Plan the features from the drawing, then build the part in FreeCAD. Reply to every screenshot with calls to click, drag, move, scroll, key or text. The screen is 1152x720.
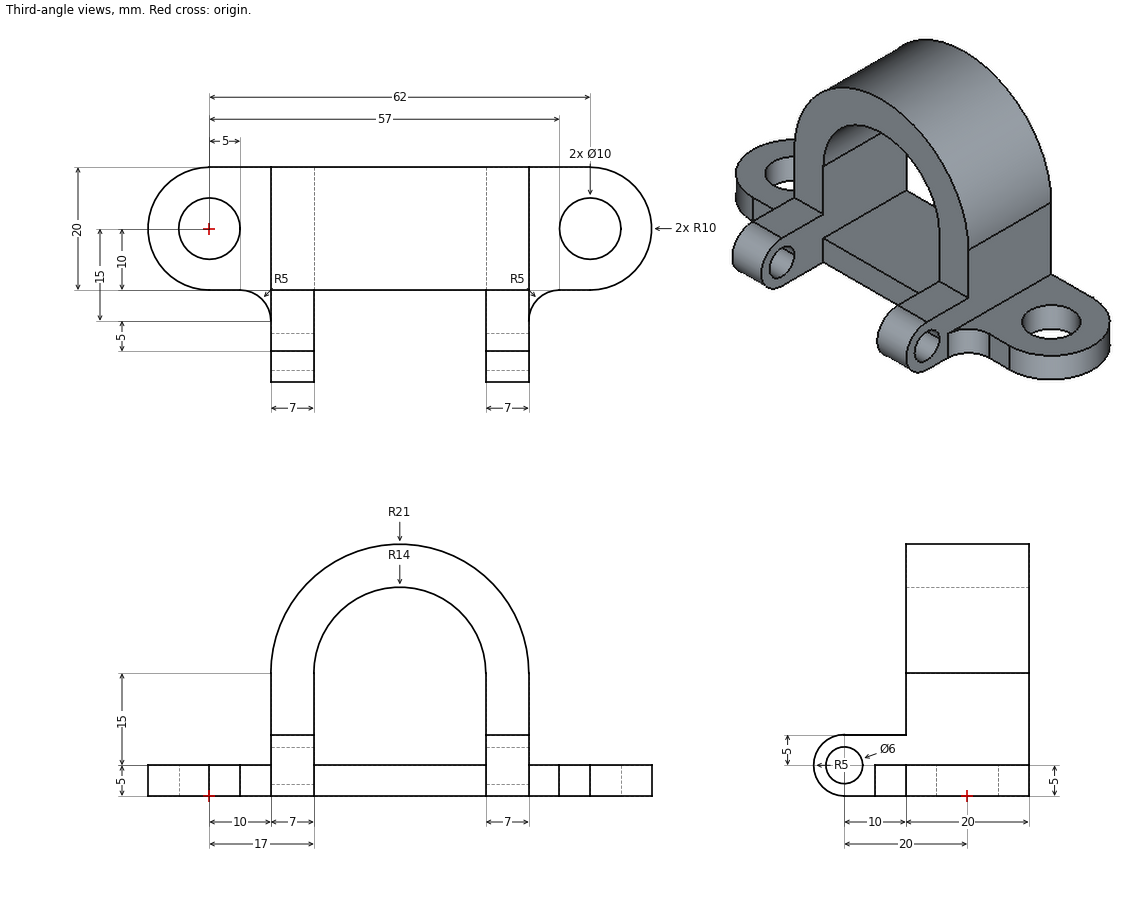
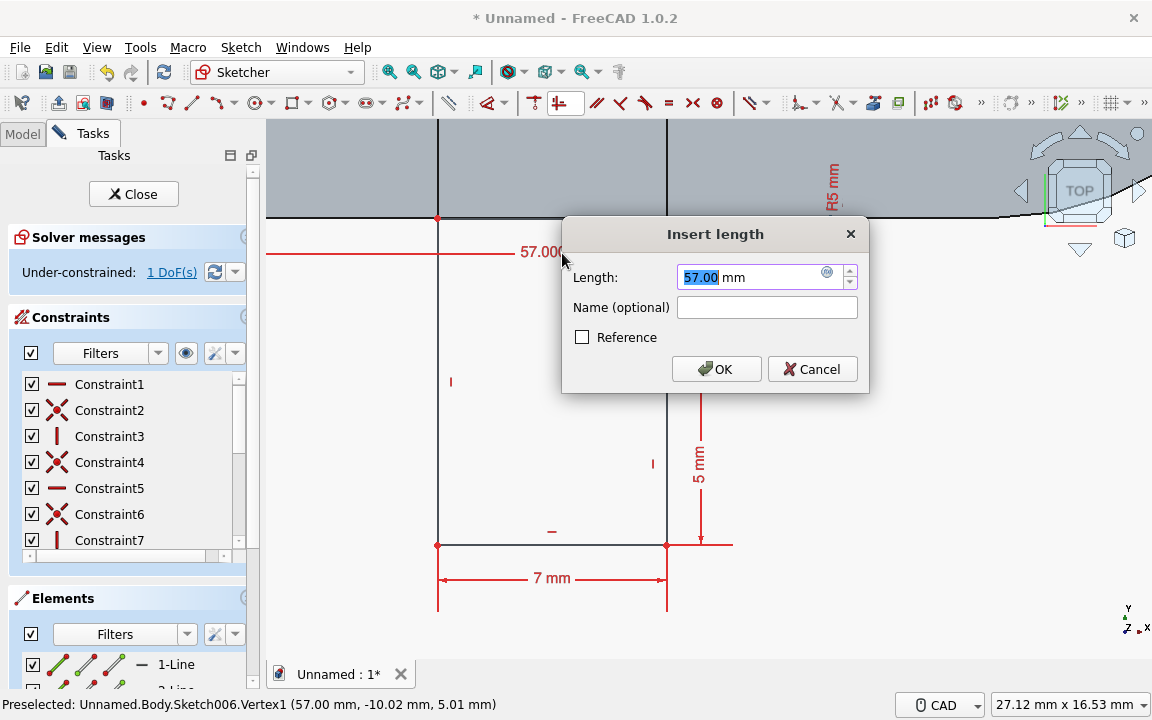
text(57)
key(Return)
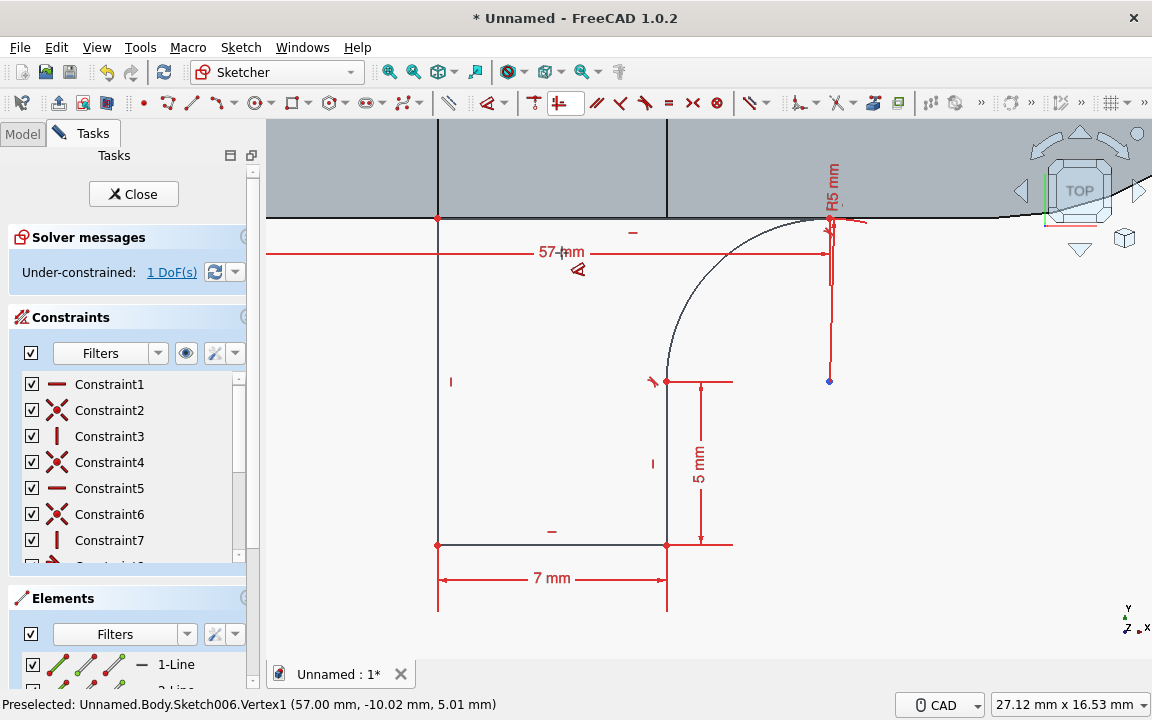
click(830, 219)
click(864, 166)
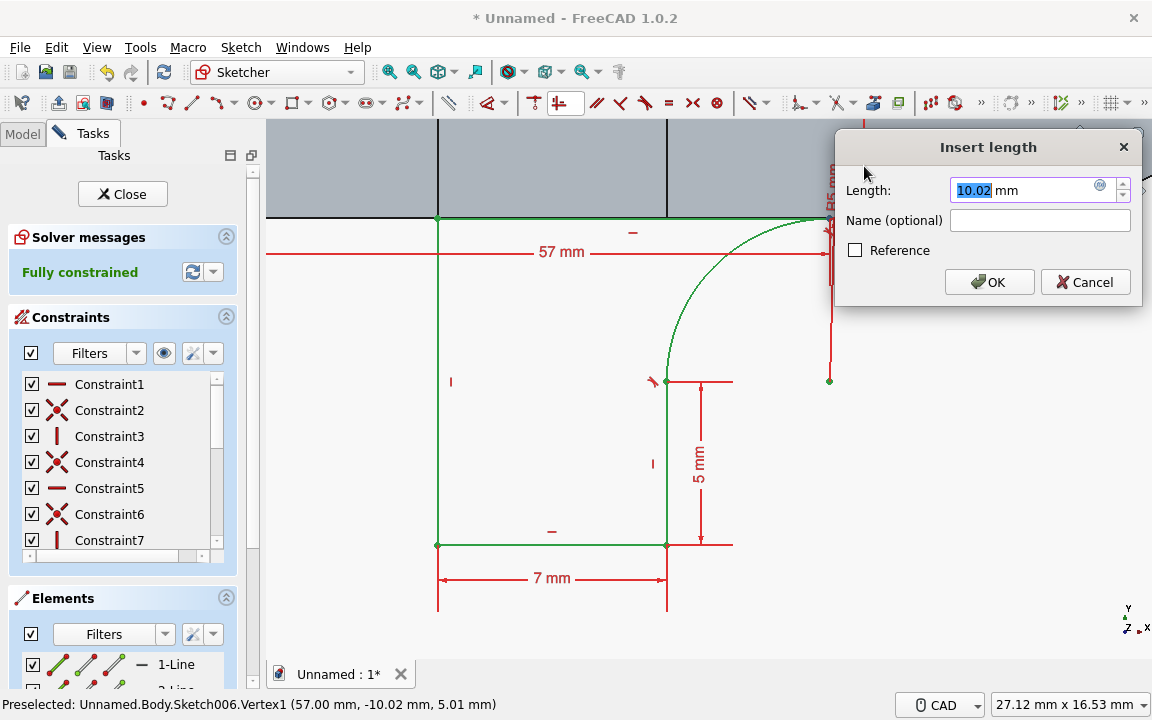
text(10)
key(Return)
key(Escape)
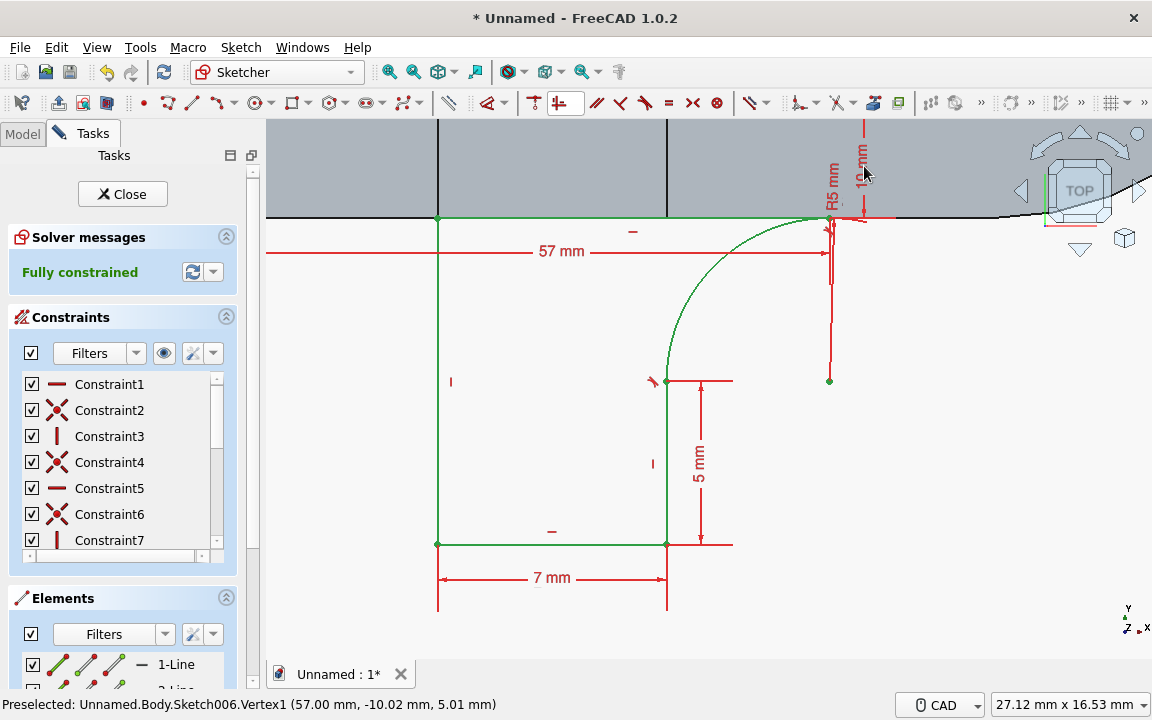
click(123, 194)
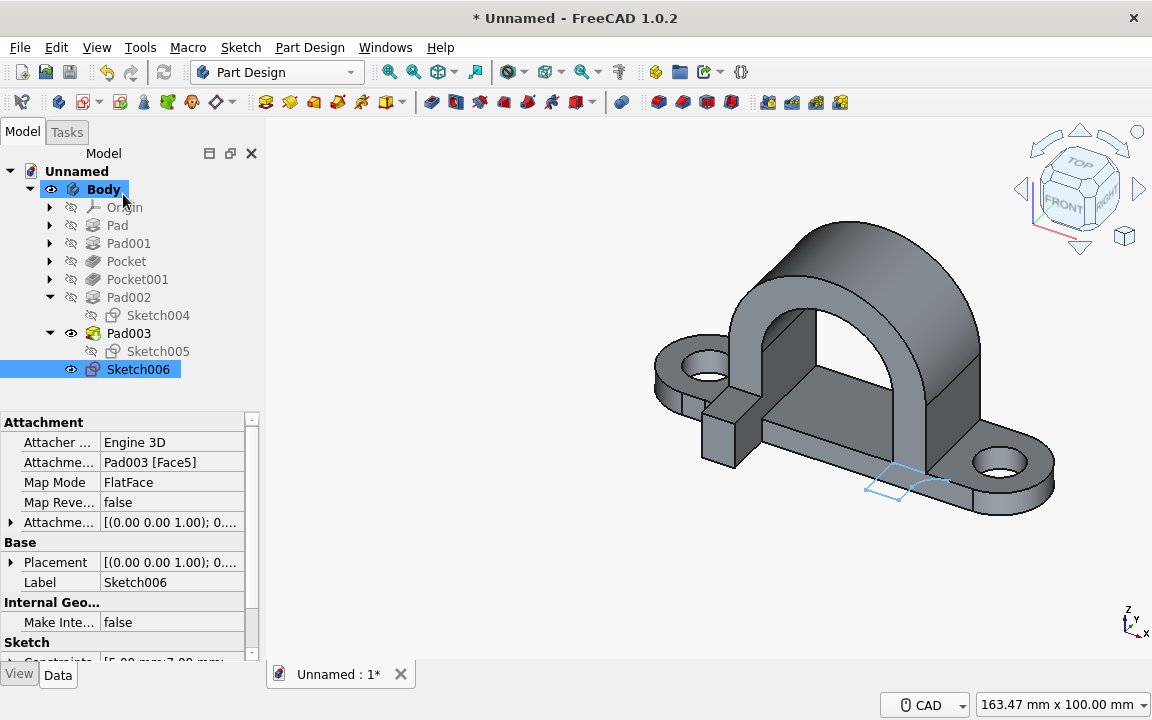
click(266, 102)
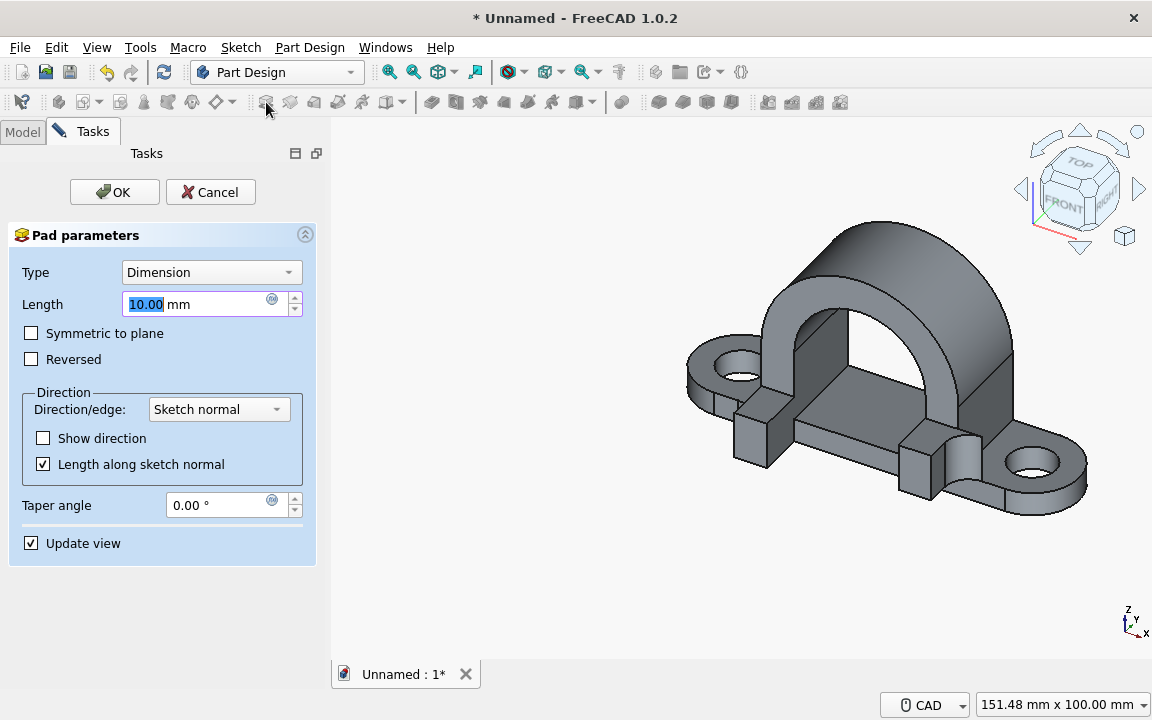
text(5)
key(Tab)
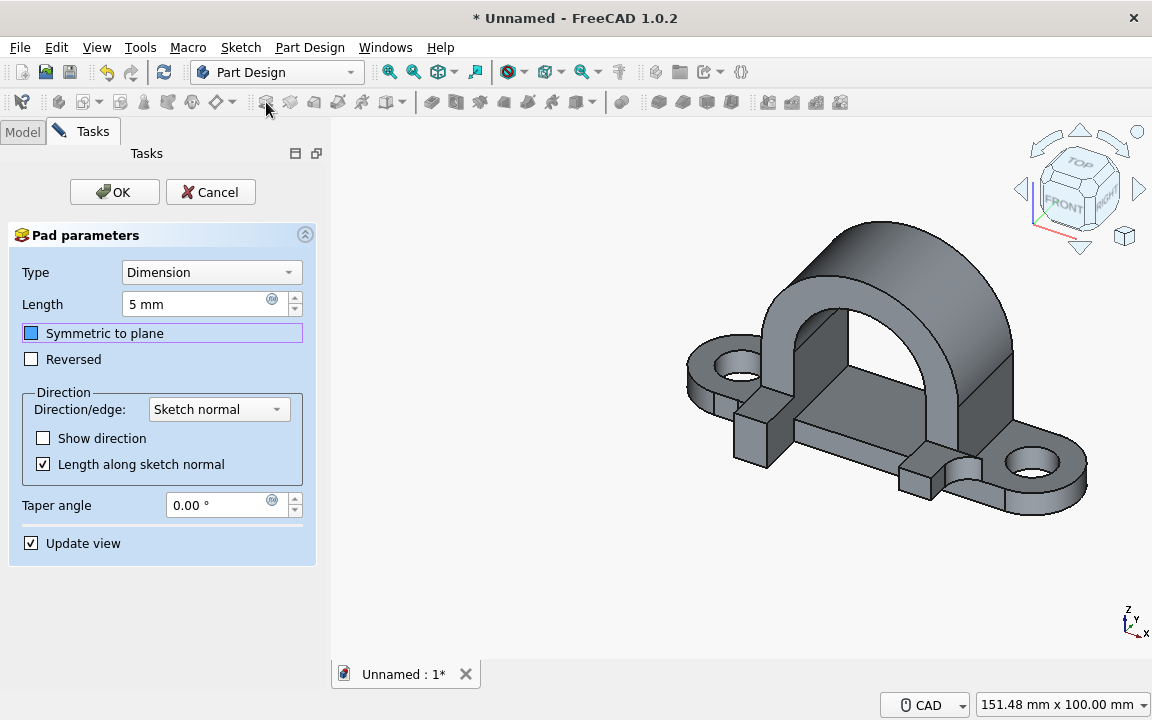
click(30, 359)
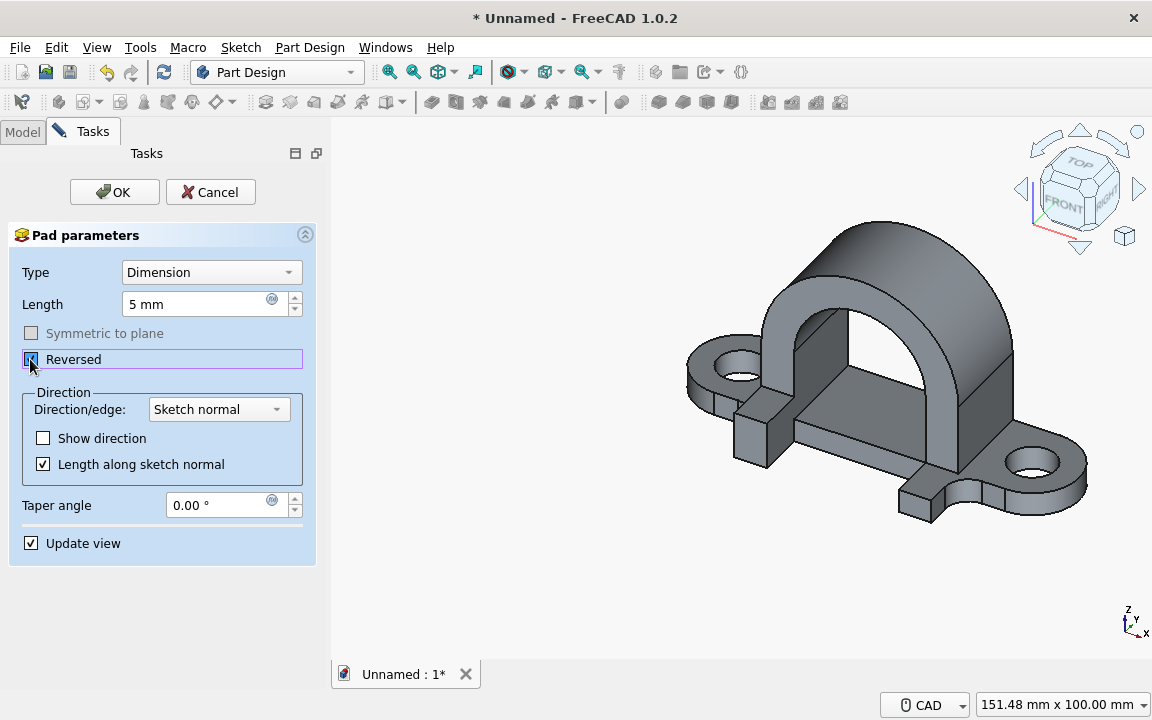
click(115, 192)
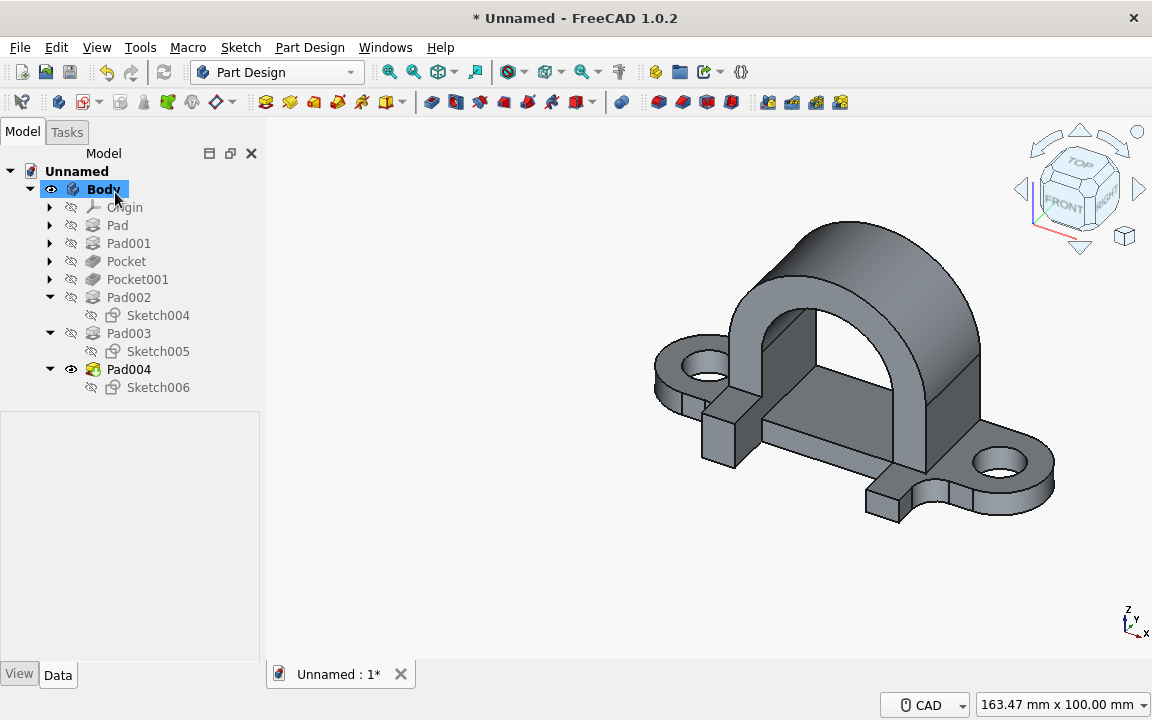
click(50, 207)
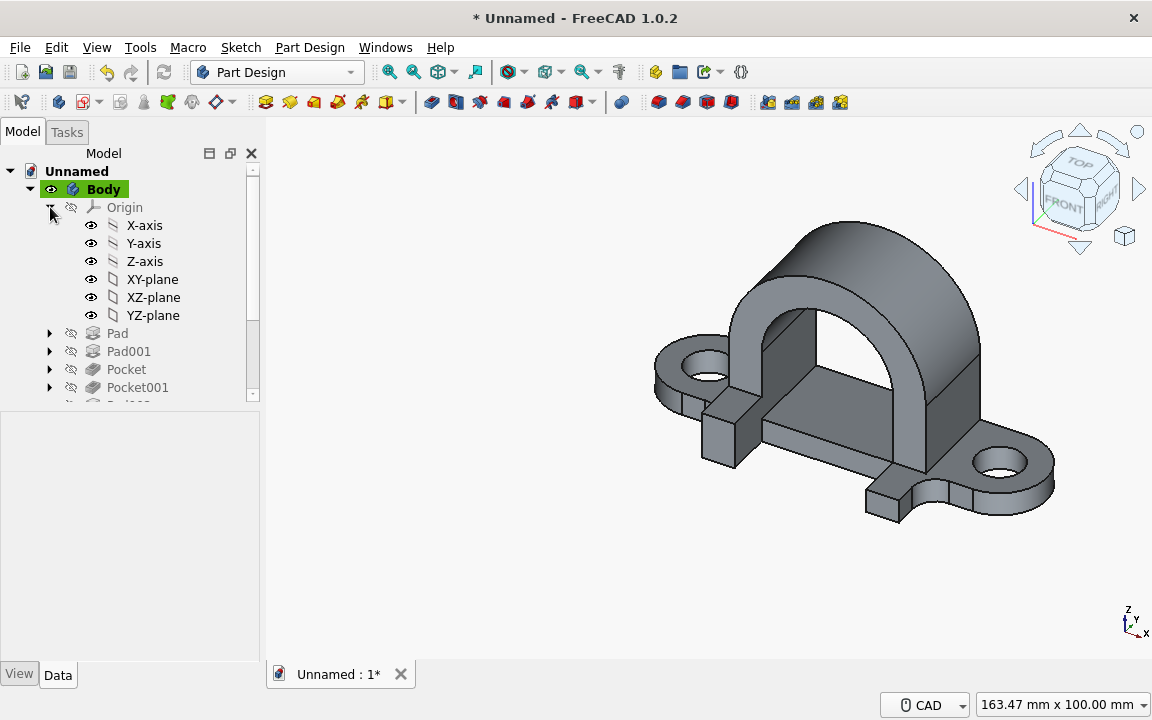
click(136, 315)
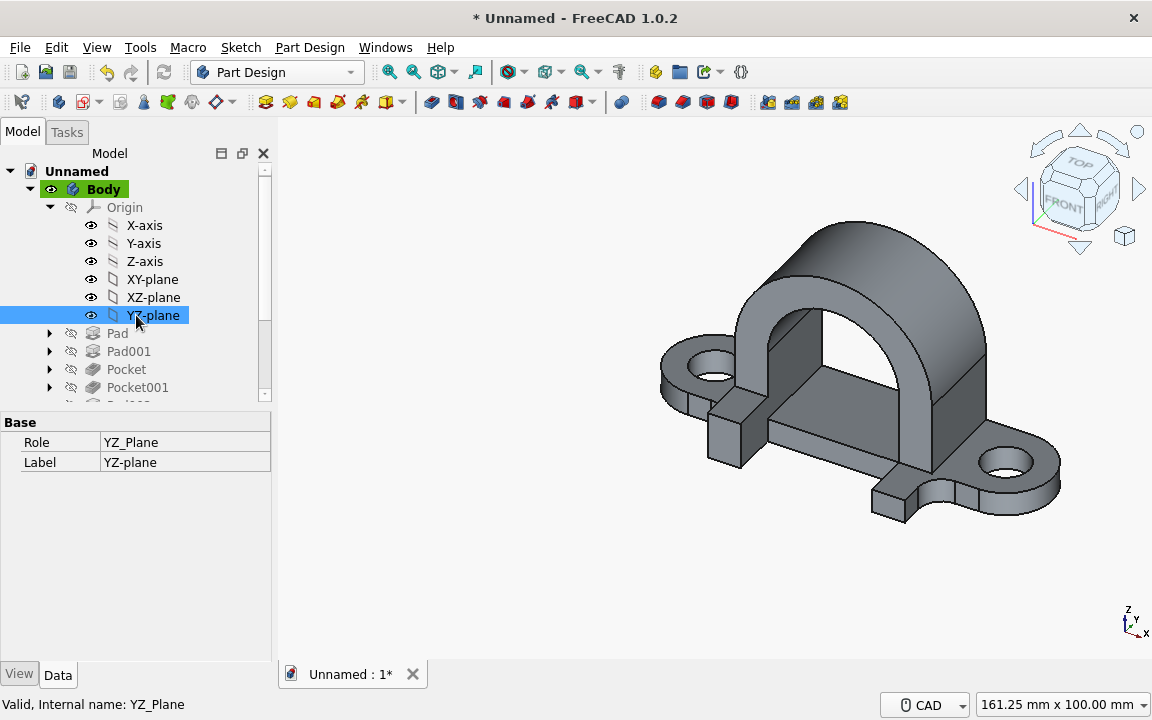
click(216, 102)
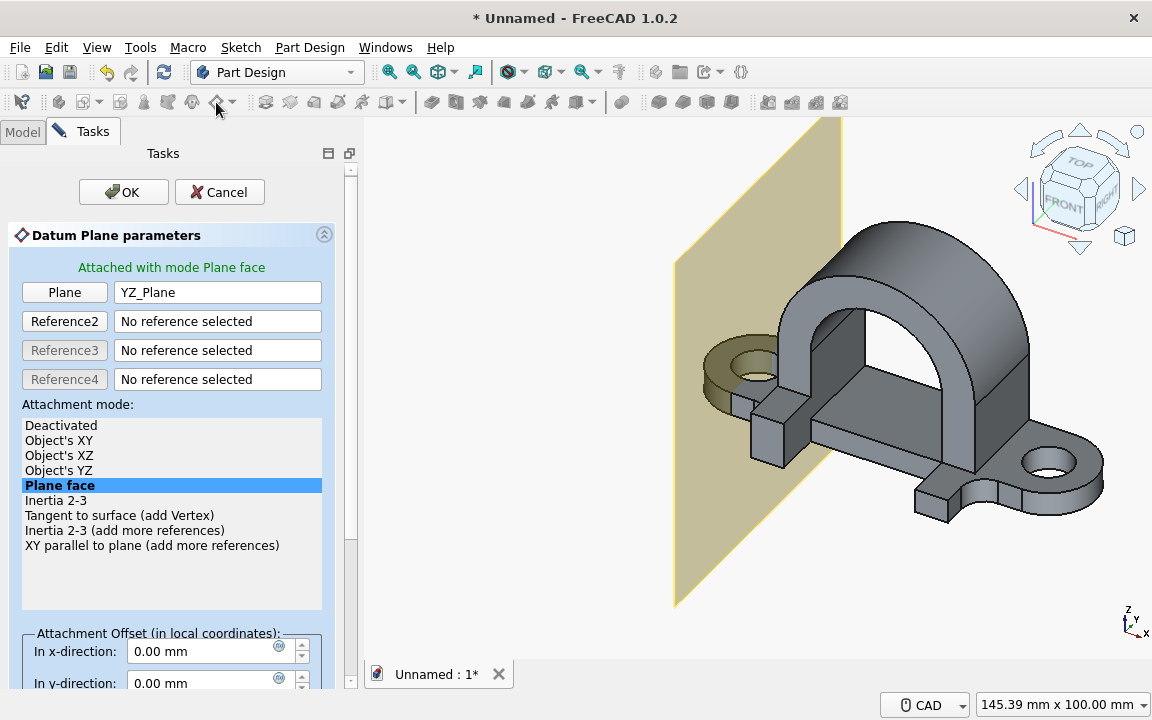
scroll(351, 426, down, 2)